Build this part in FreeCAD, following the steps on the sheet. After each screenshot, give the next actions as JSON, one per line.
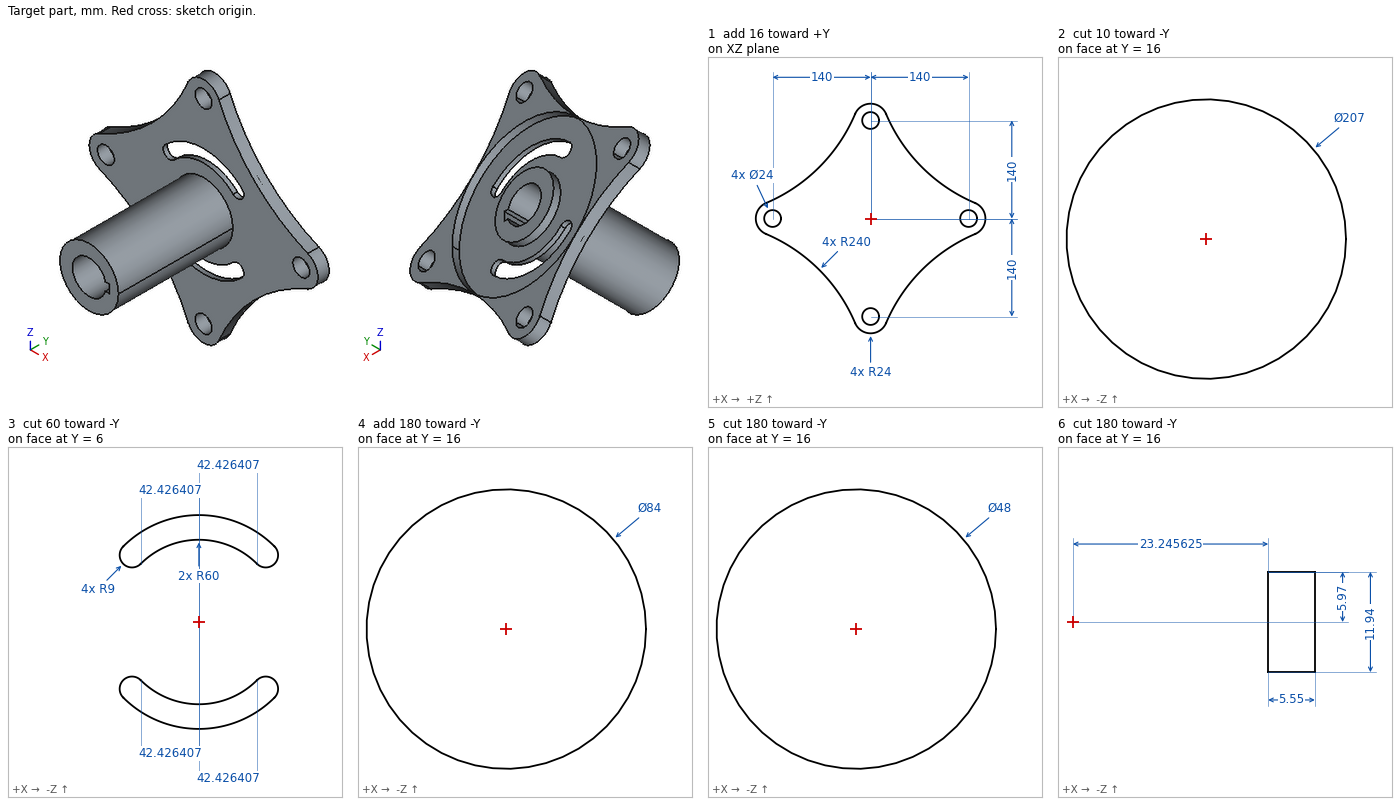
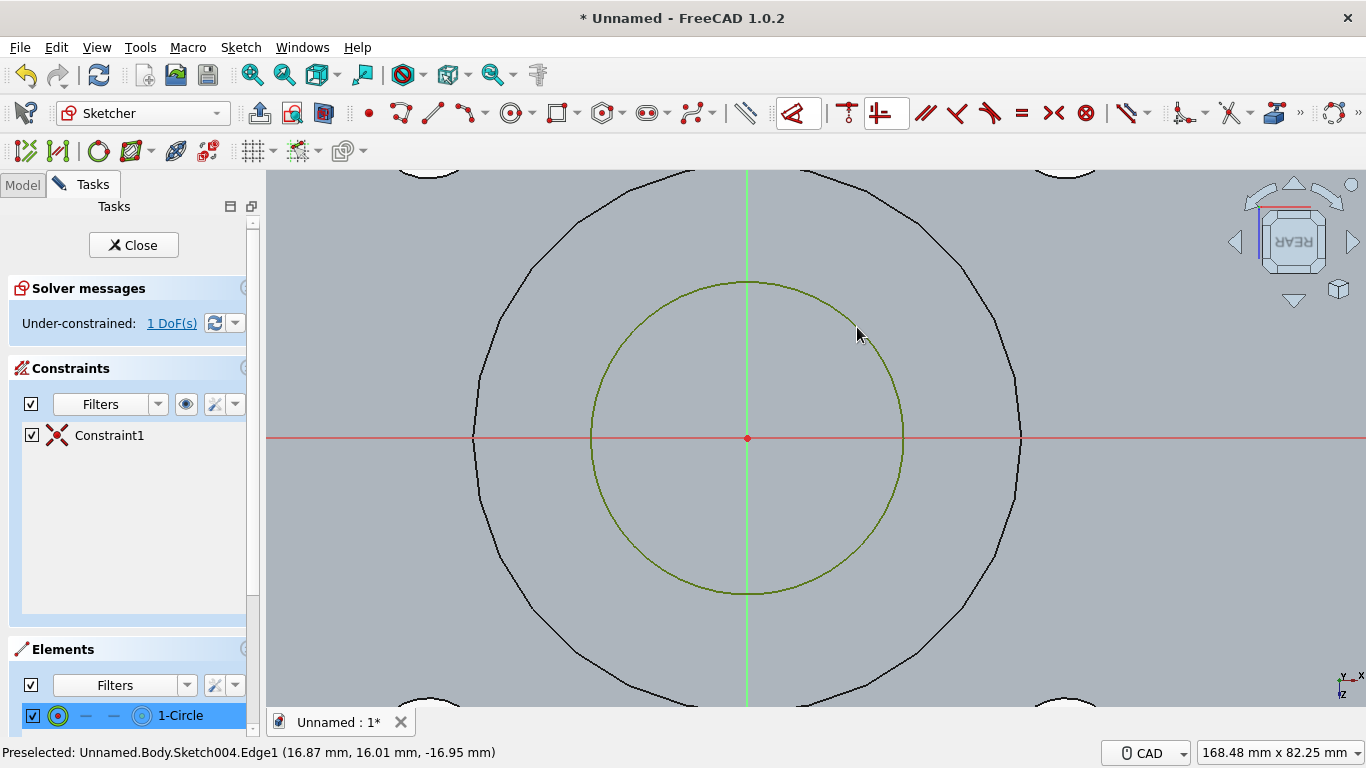
{"action": "left_click", "coordinate": [816, 114]}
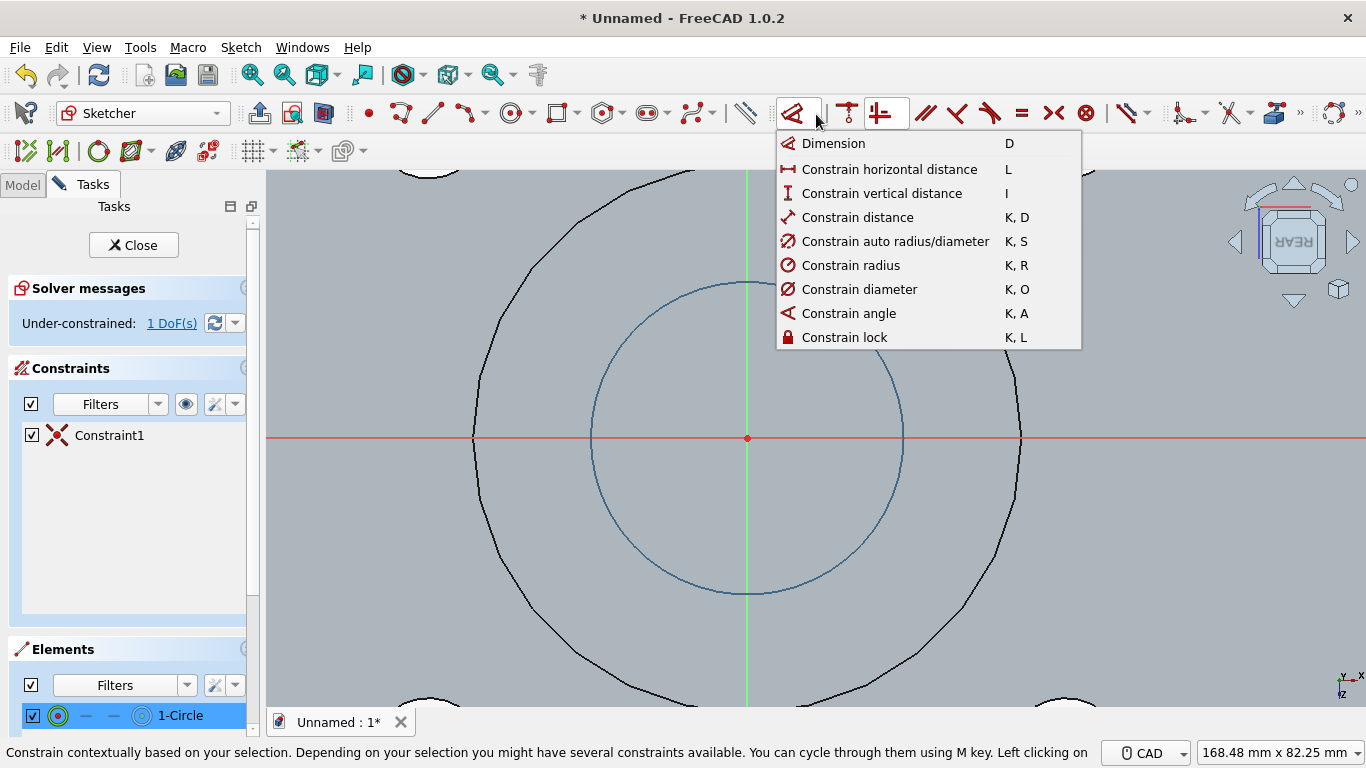
{"action": "left_click", "coordinate": [929, 289]}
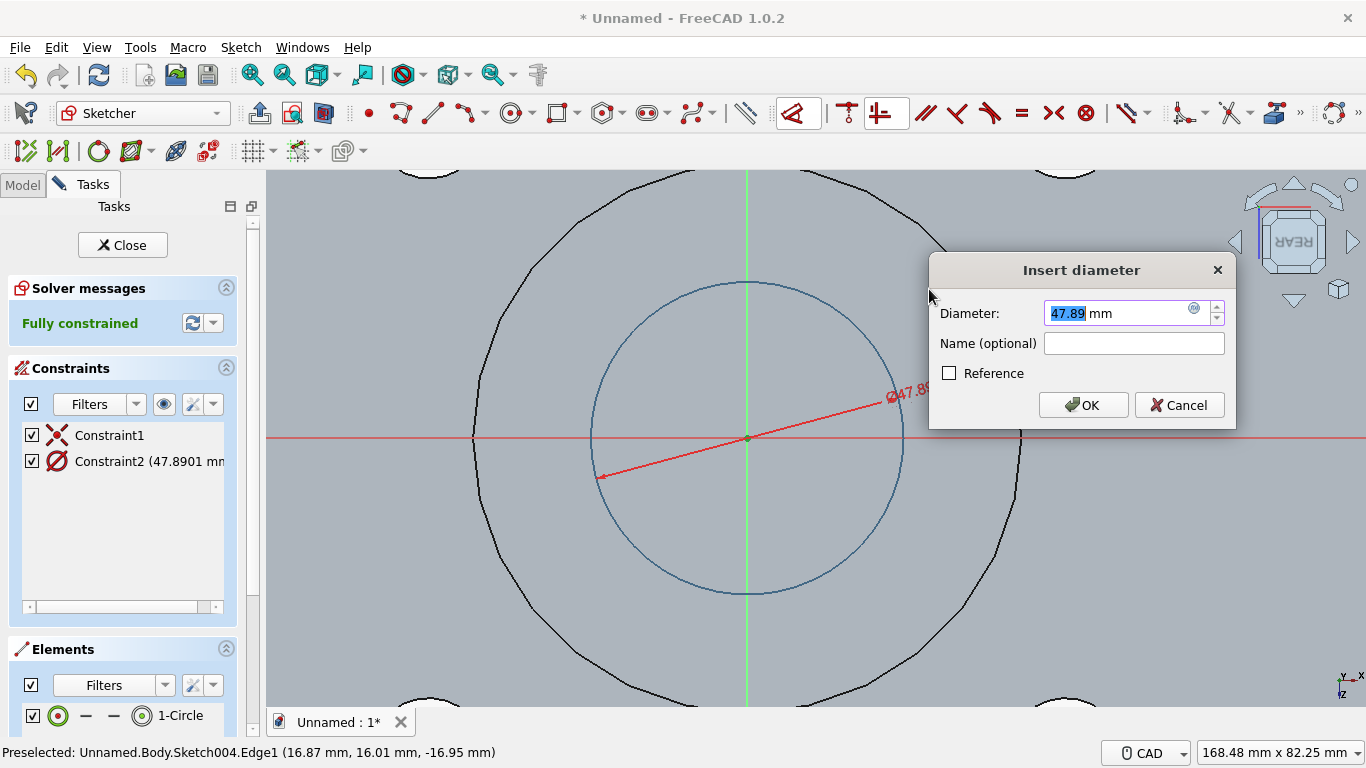
{"action": "type", "text": "48"}
{"action": "key", "text": "Return"}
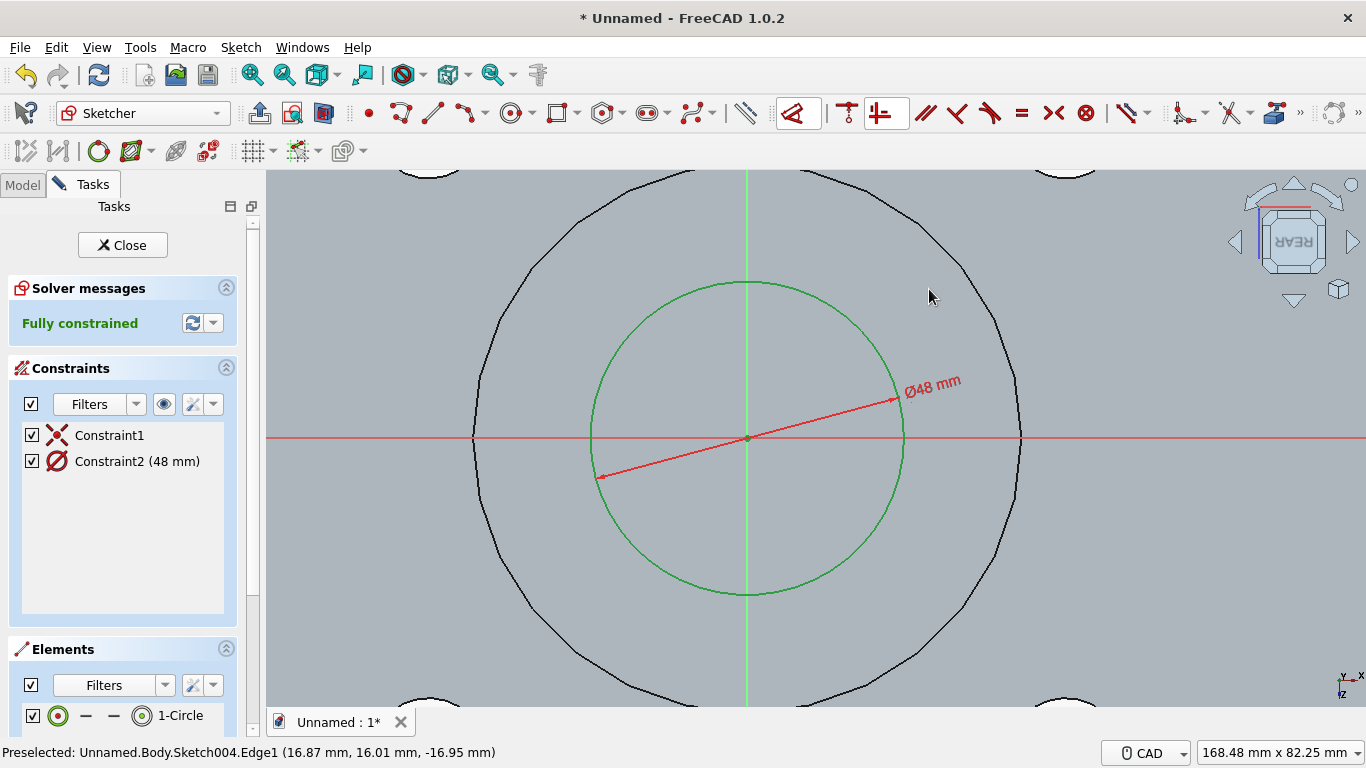
{"action": "left_click", "coordinate": [123, 245]}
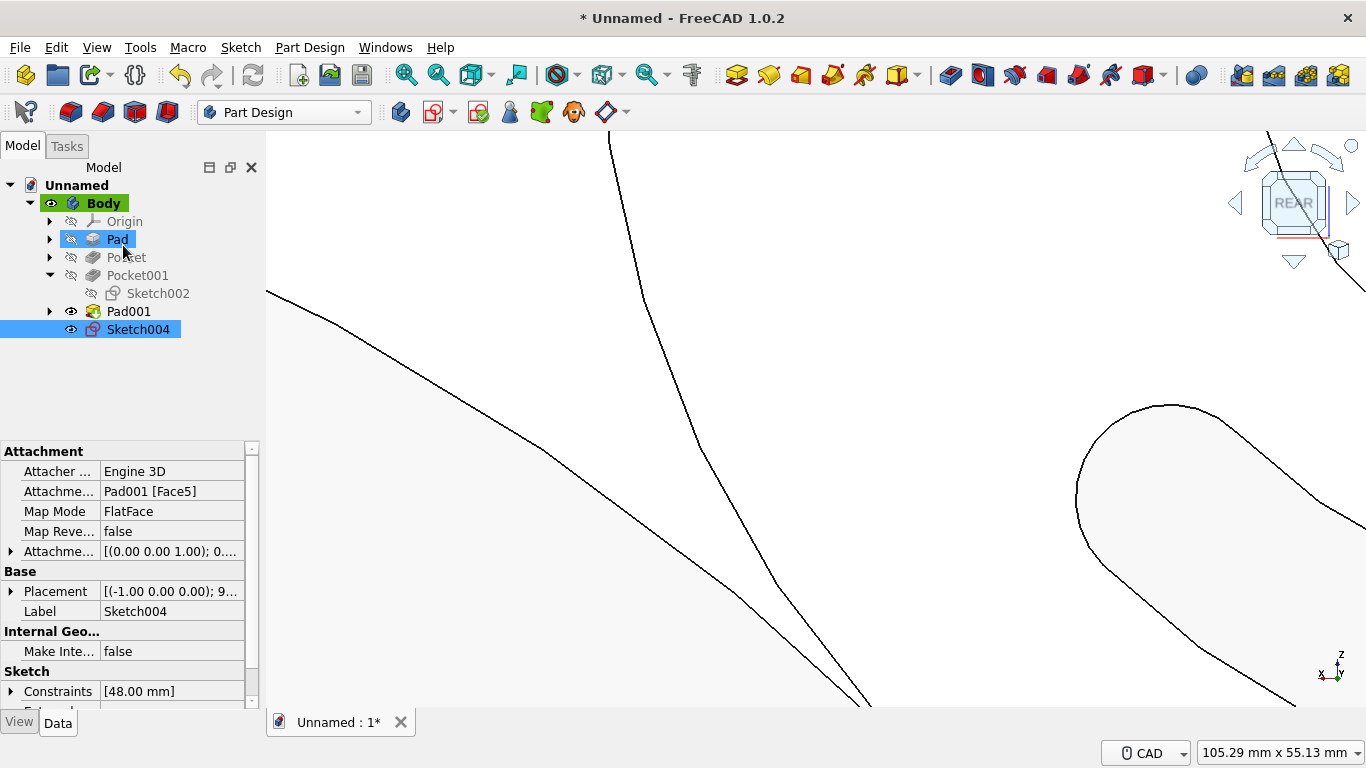
{"action": "left_click", "coordinate": [952, 76]}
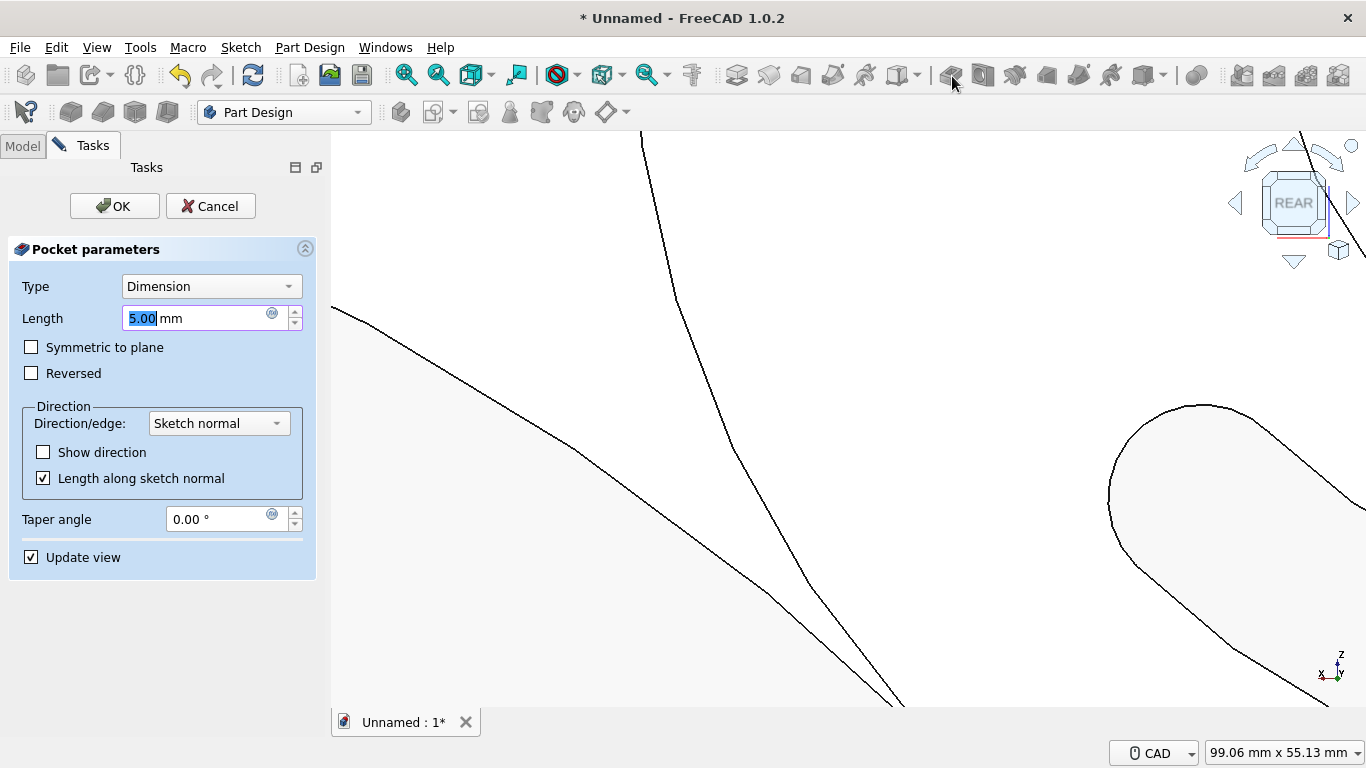
{"action": "type", "text": "180"}
{"action": "key", "text": "Tab"}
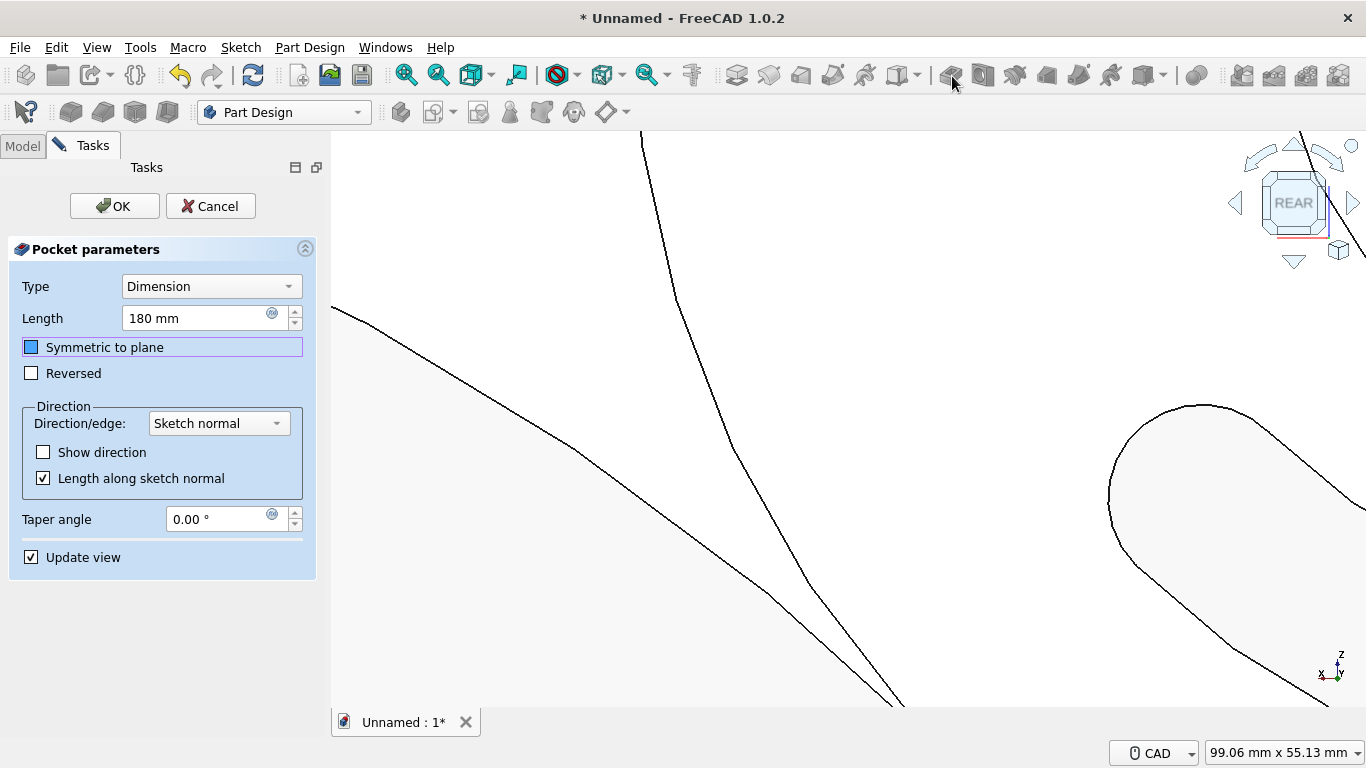
{"action": "left_click", "coordinate": [115, 206]}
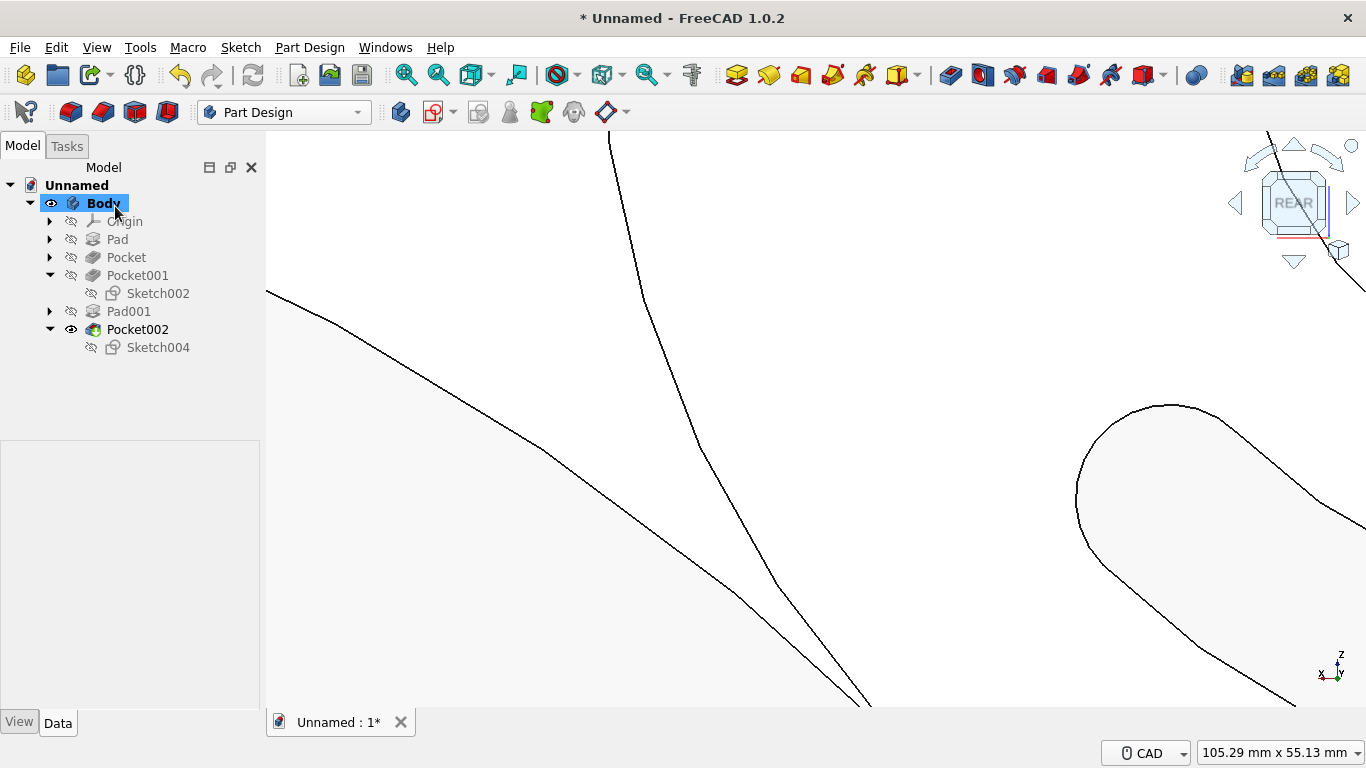
{"action": "left_click", "coordinate": [408, 76]}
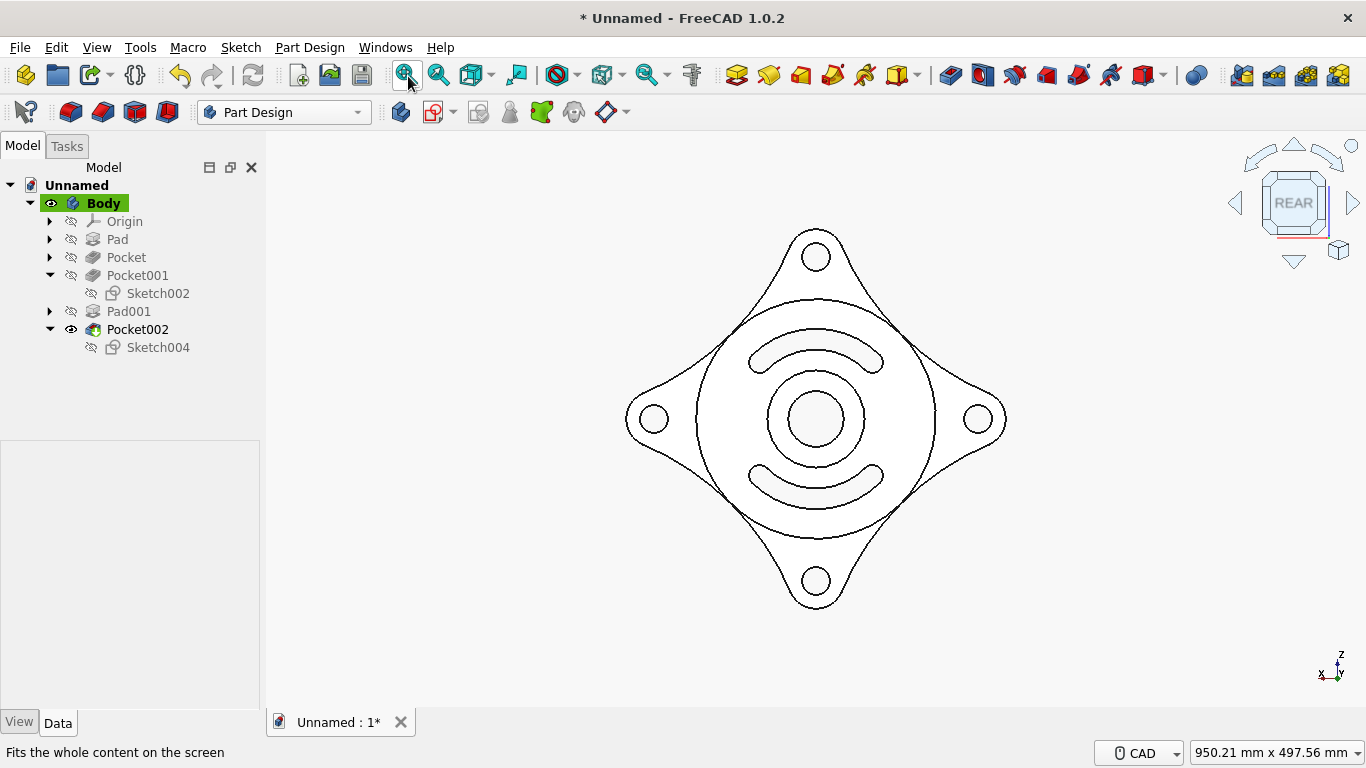
{"action": "scroll", "coordinate": [708, 472], "scroll_direction": "up", "scroll_amount": 11}